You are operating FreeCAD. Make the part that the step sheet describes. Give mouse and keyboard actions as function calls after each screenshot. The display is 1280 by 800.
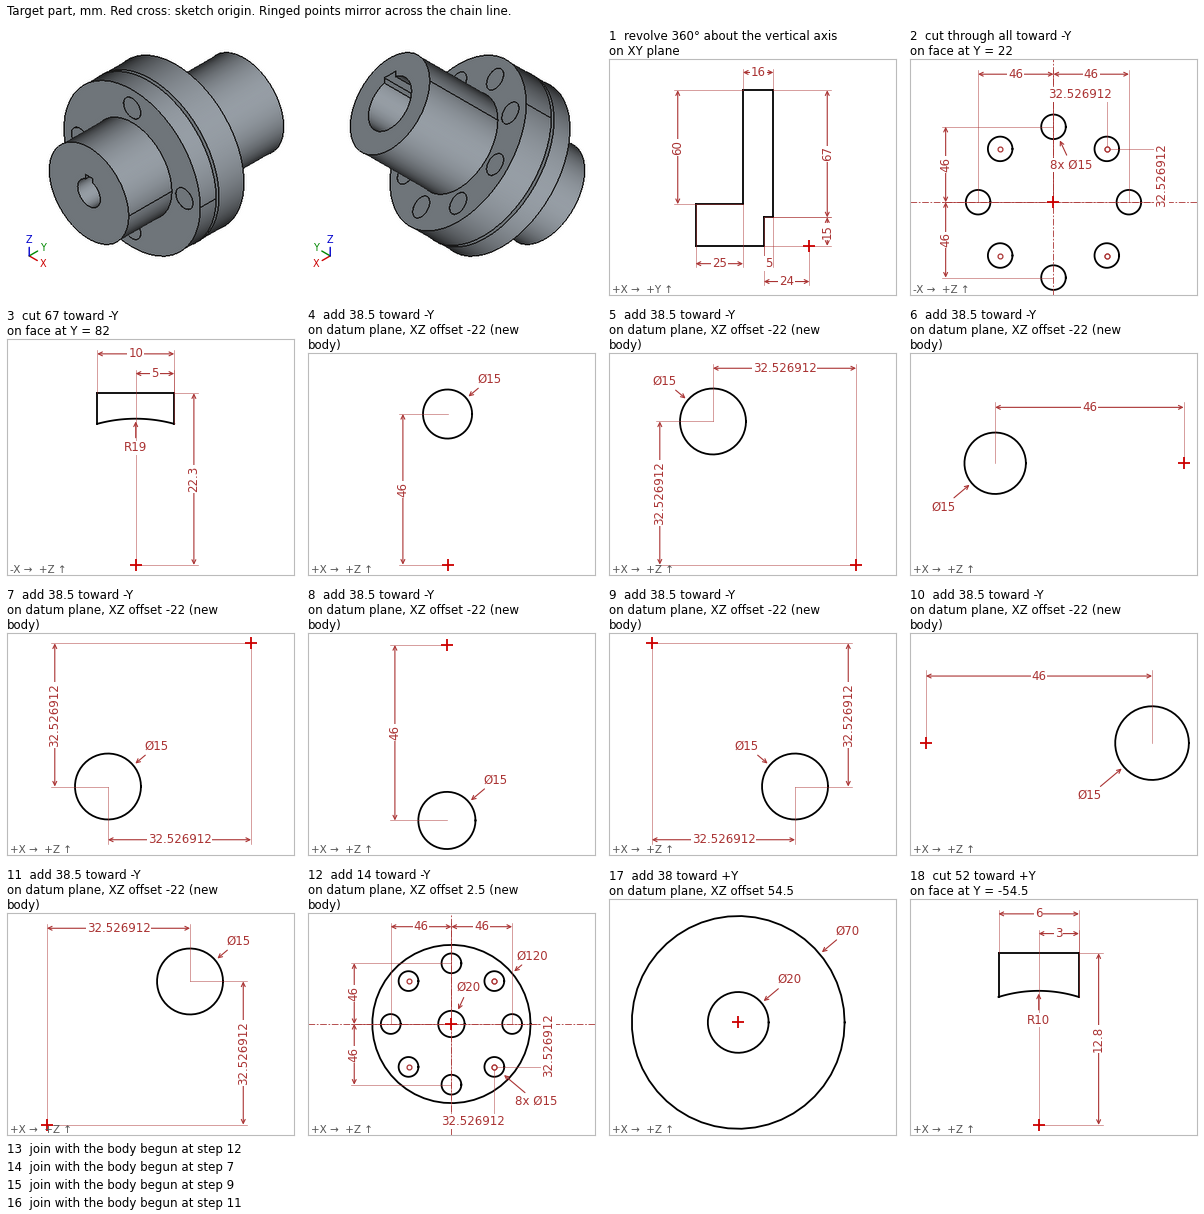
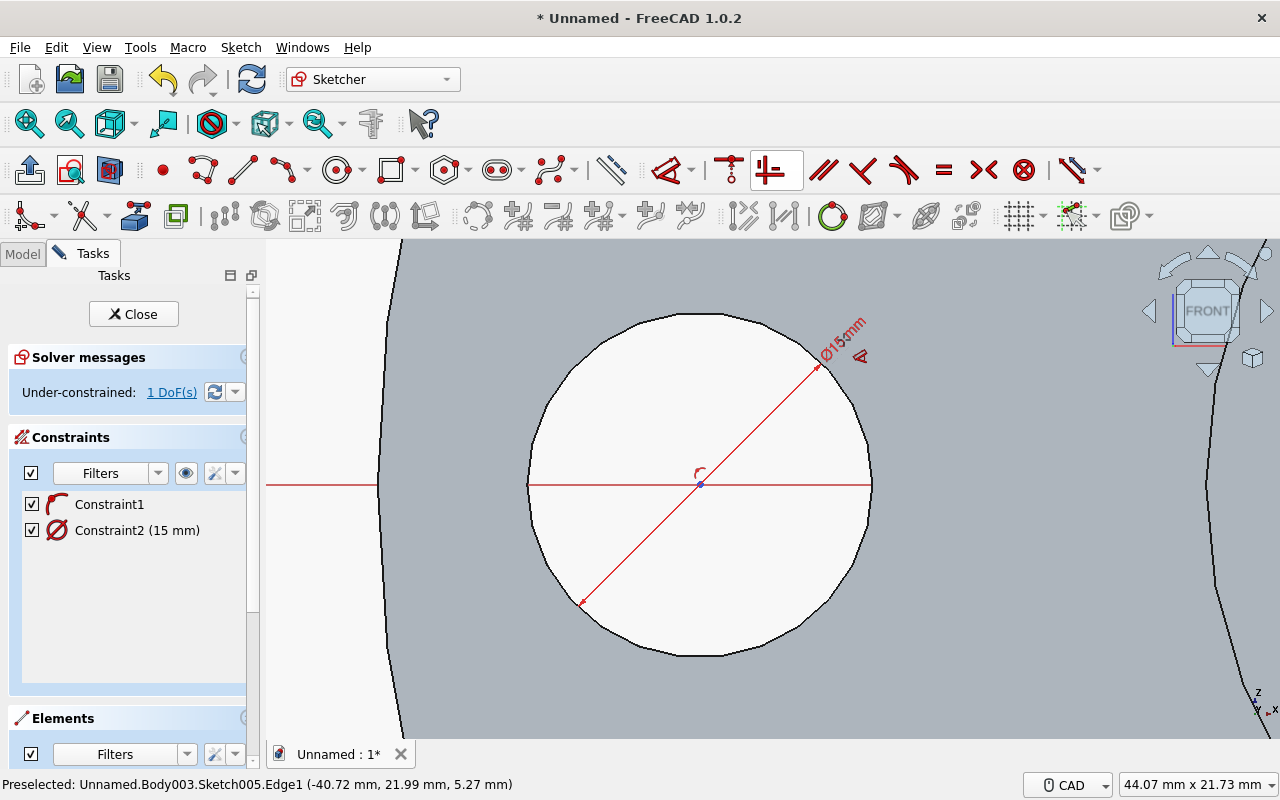
click(700, 485)
click(908, 519)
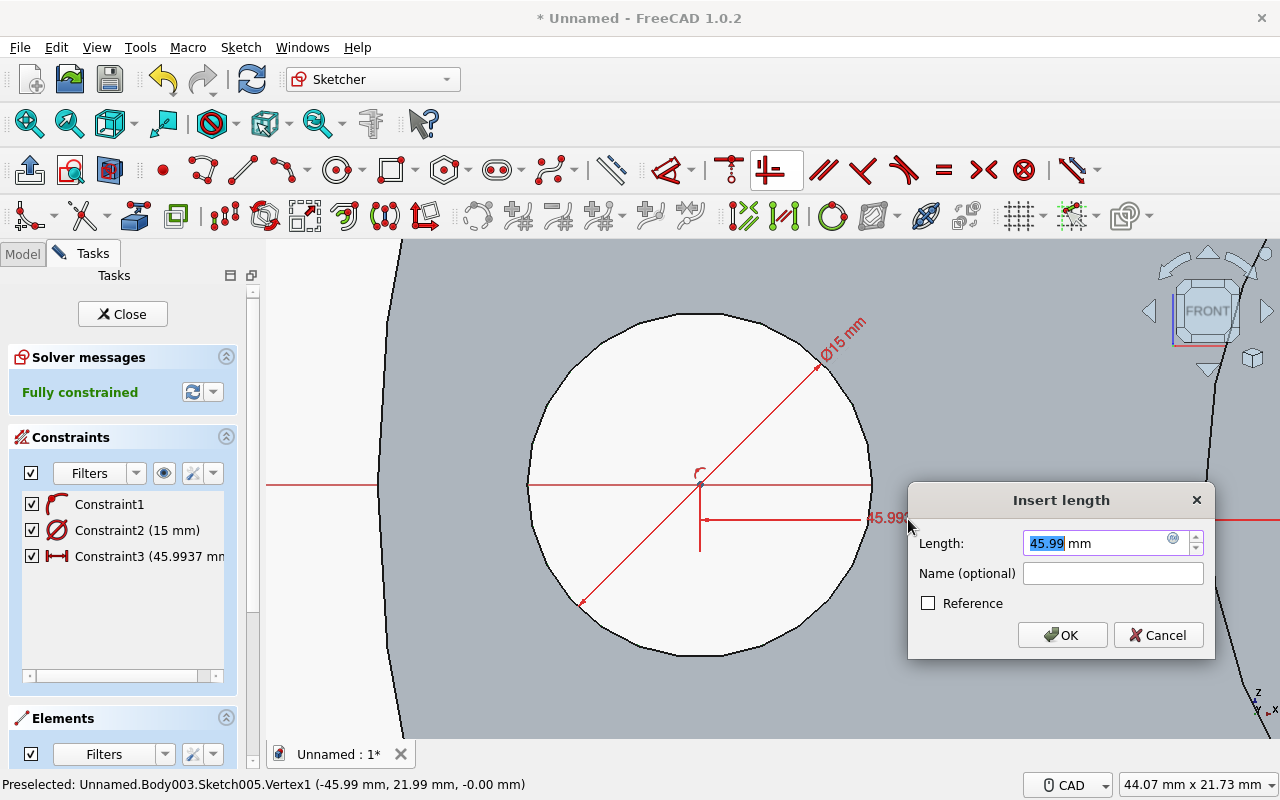
text(46)
key(Return)
key(Escape)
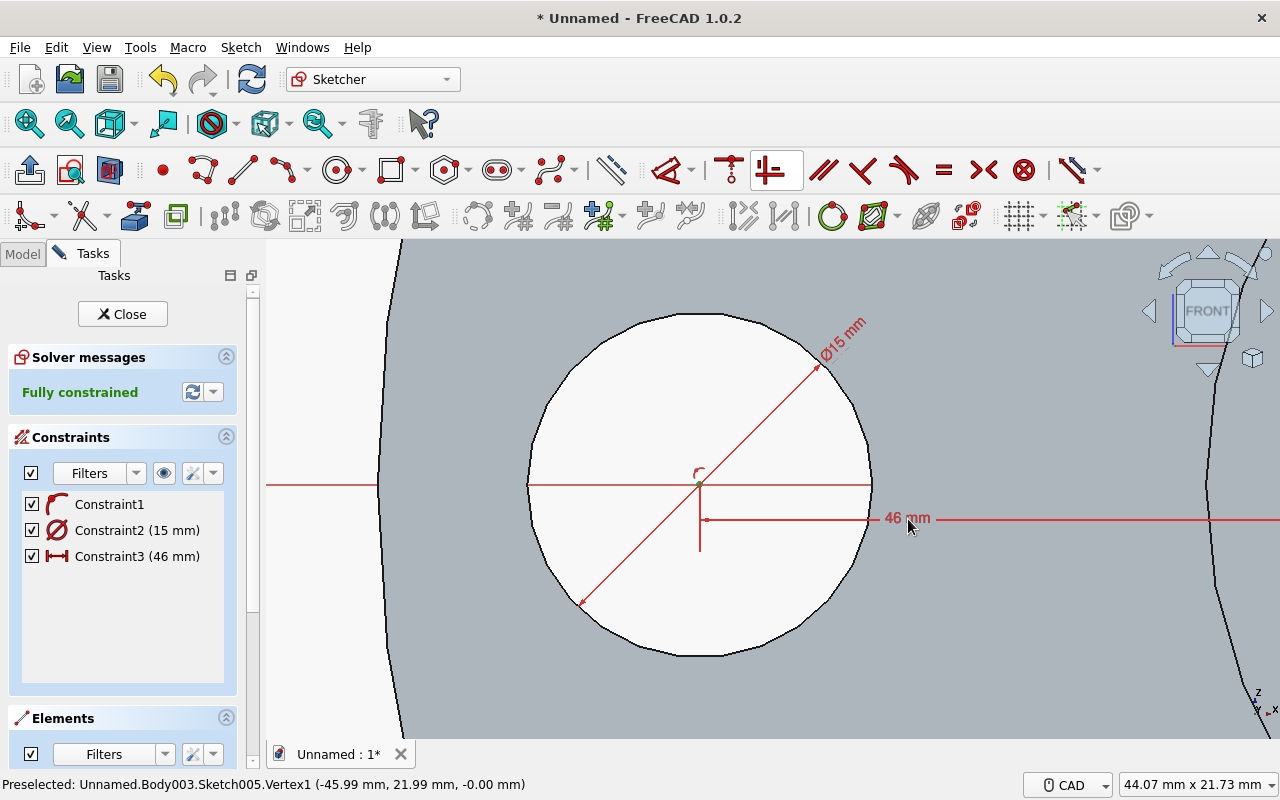
click(123, 314)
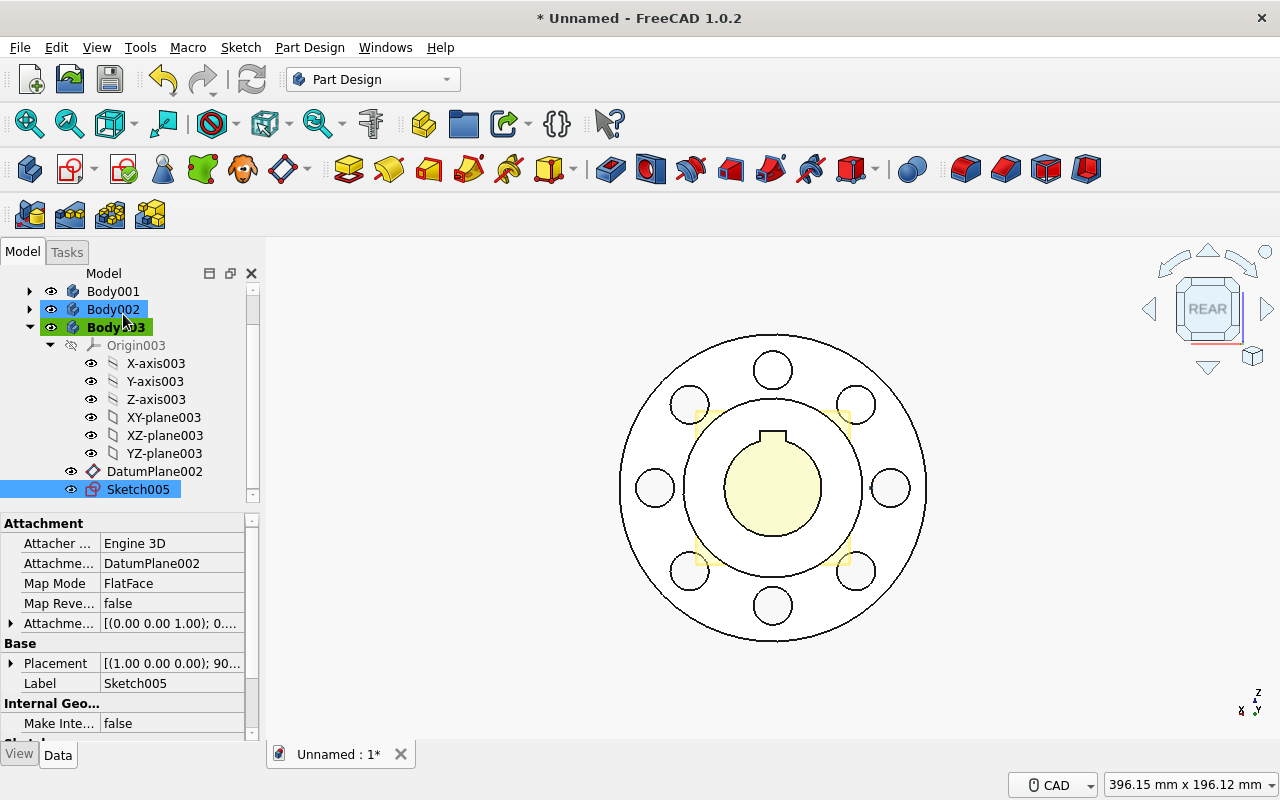
click(350, 170)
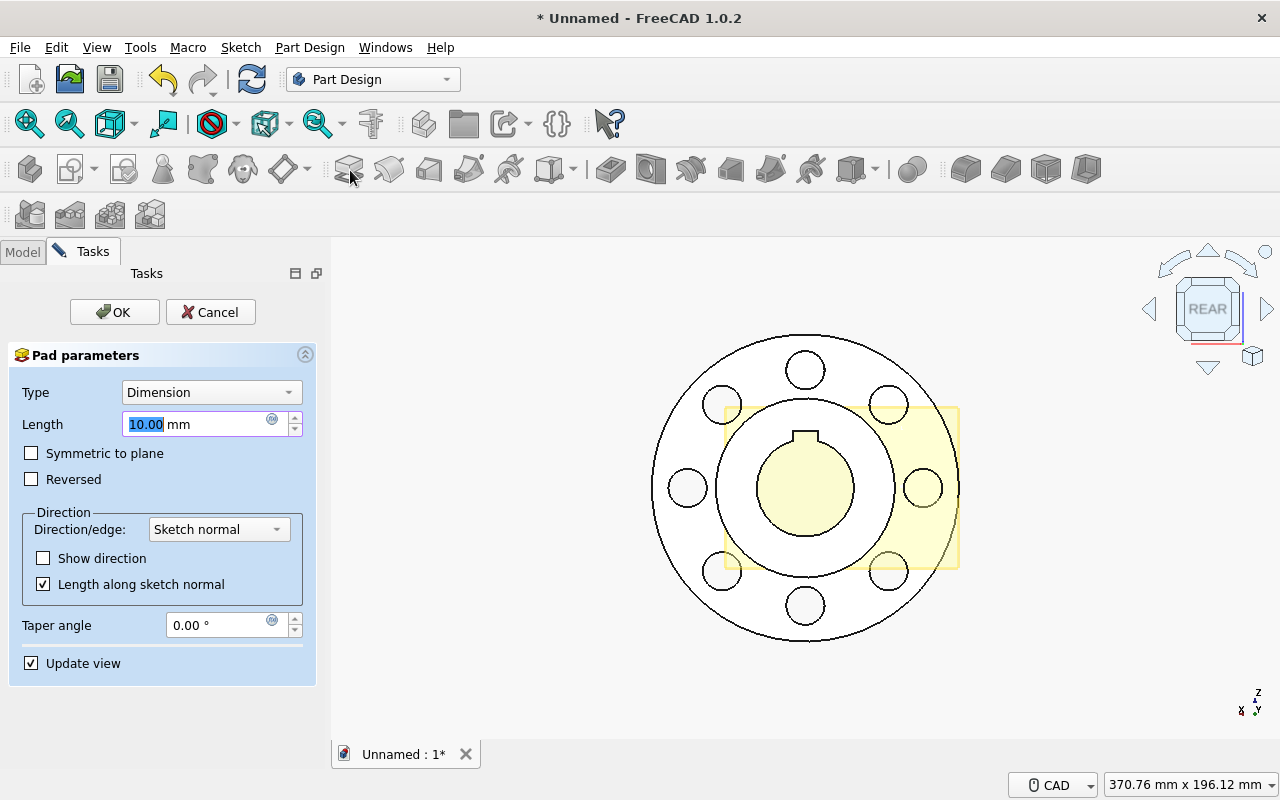
text(38.5)
key(Tab)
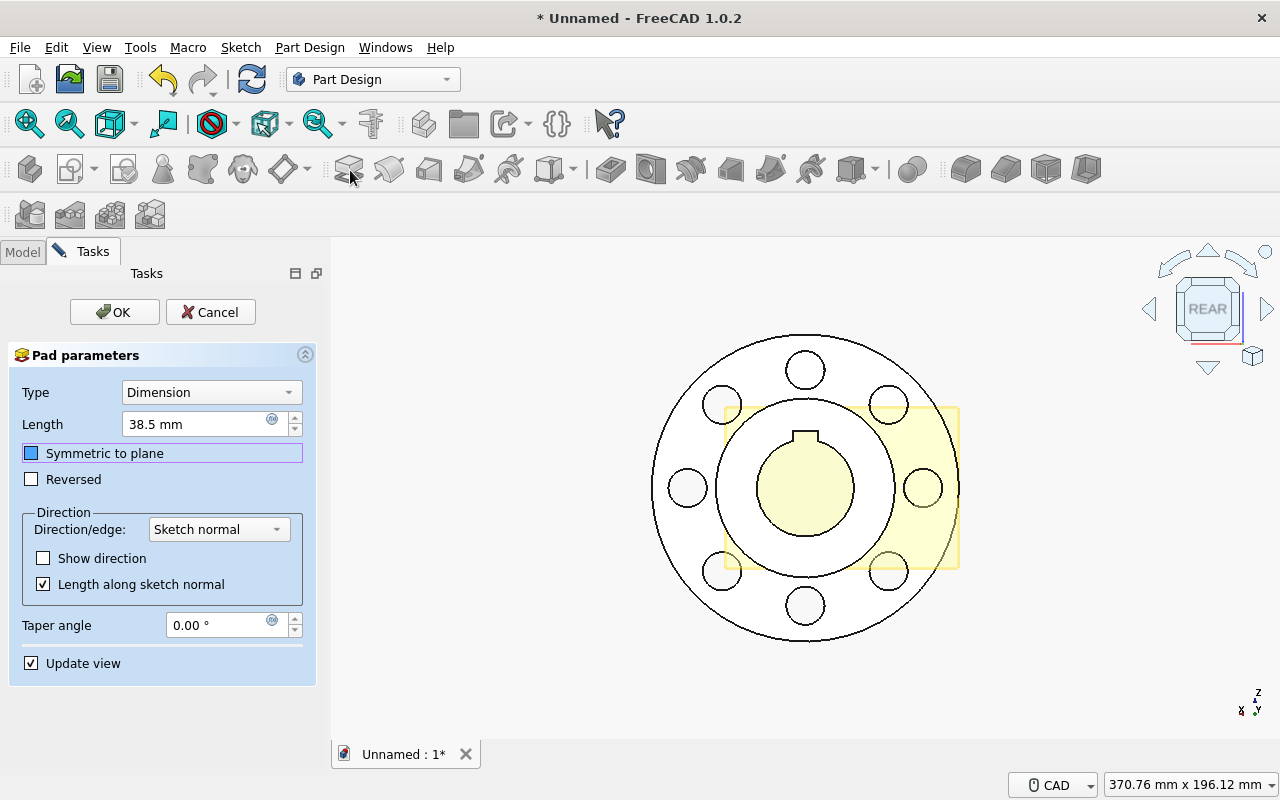
click(115, 312)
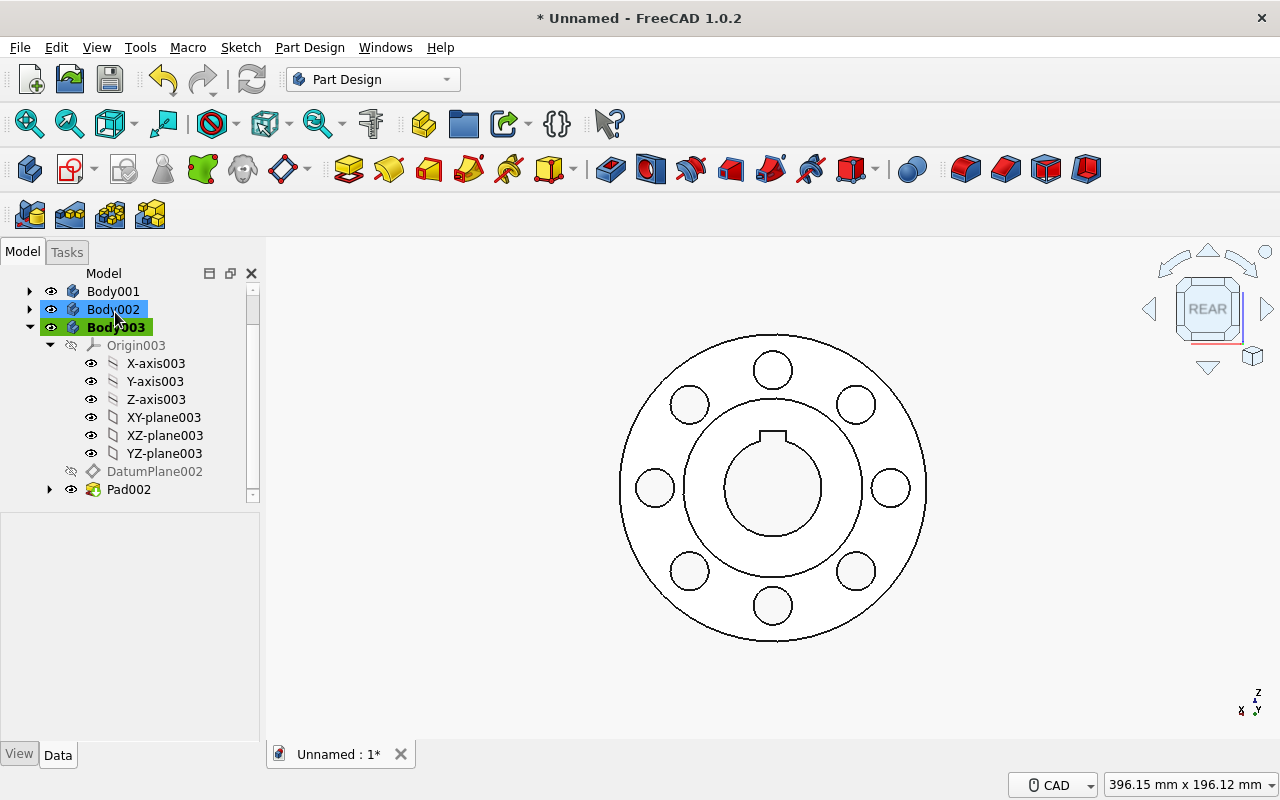
click(30, 124)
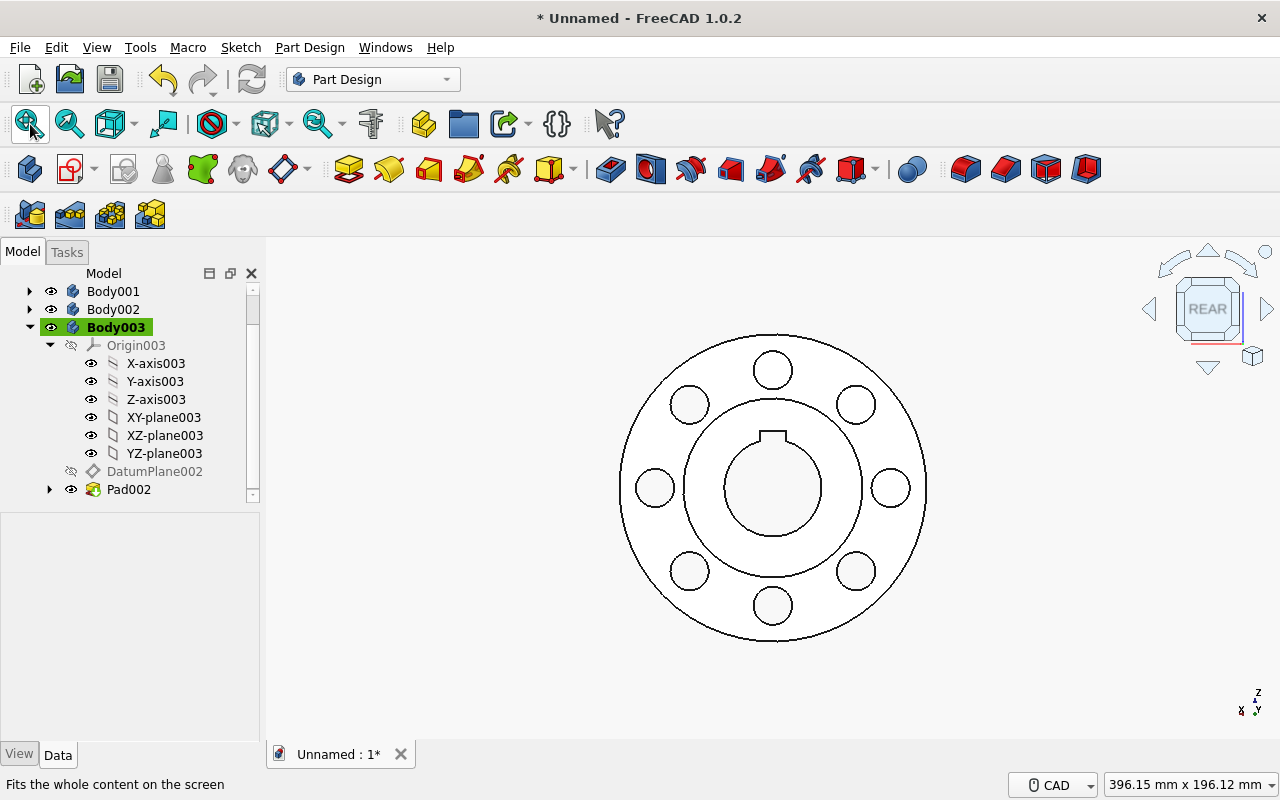
click(30, 170)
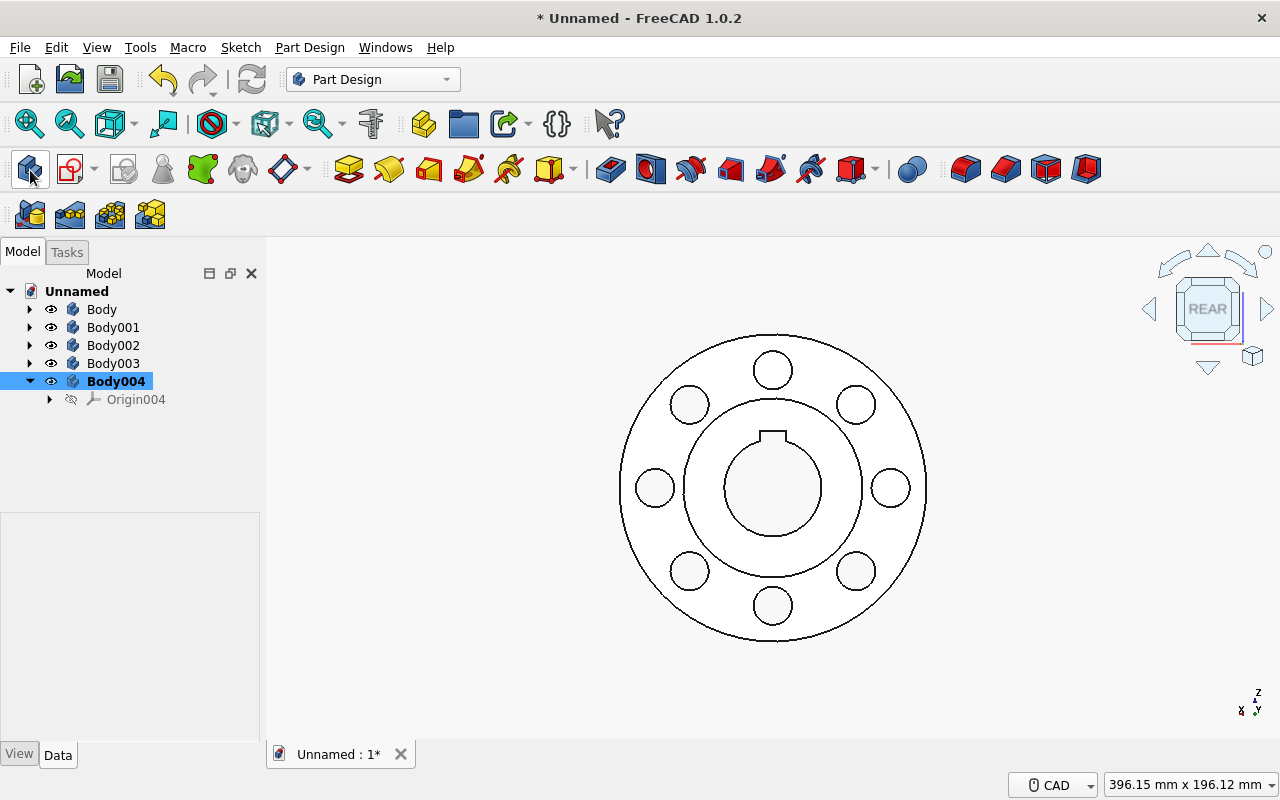
click(50, 399)